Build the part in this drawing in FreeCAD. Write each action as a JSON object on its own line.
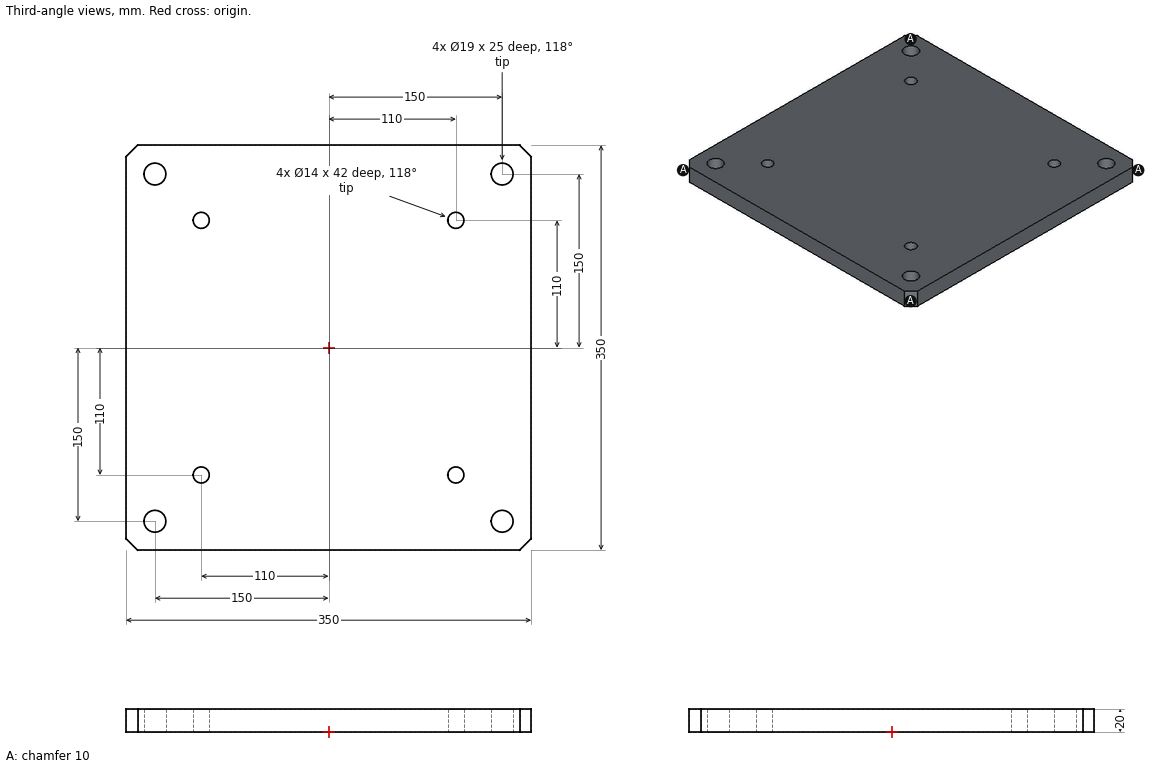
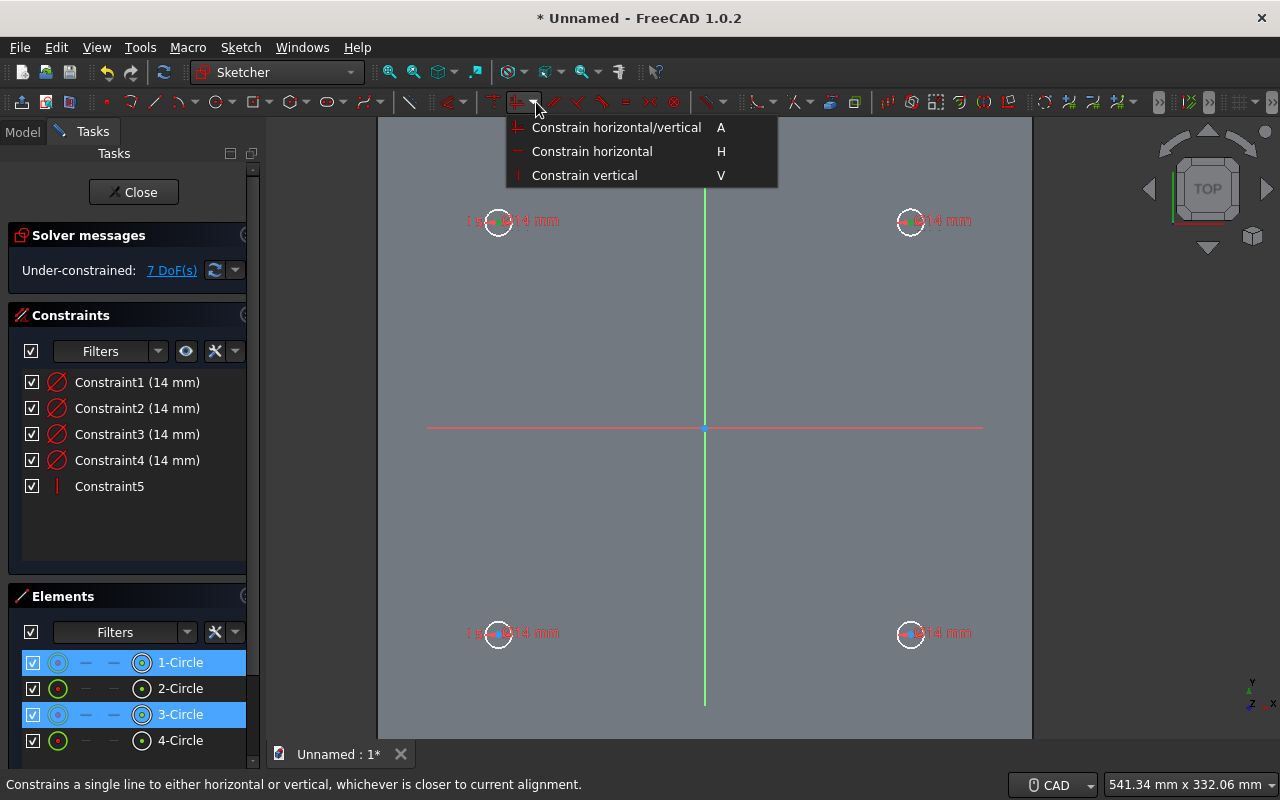
{"action": "left_click", "coordinate": [642, 151]}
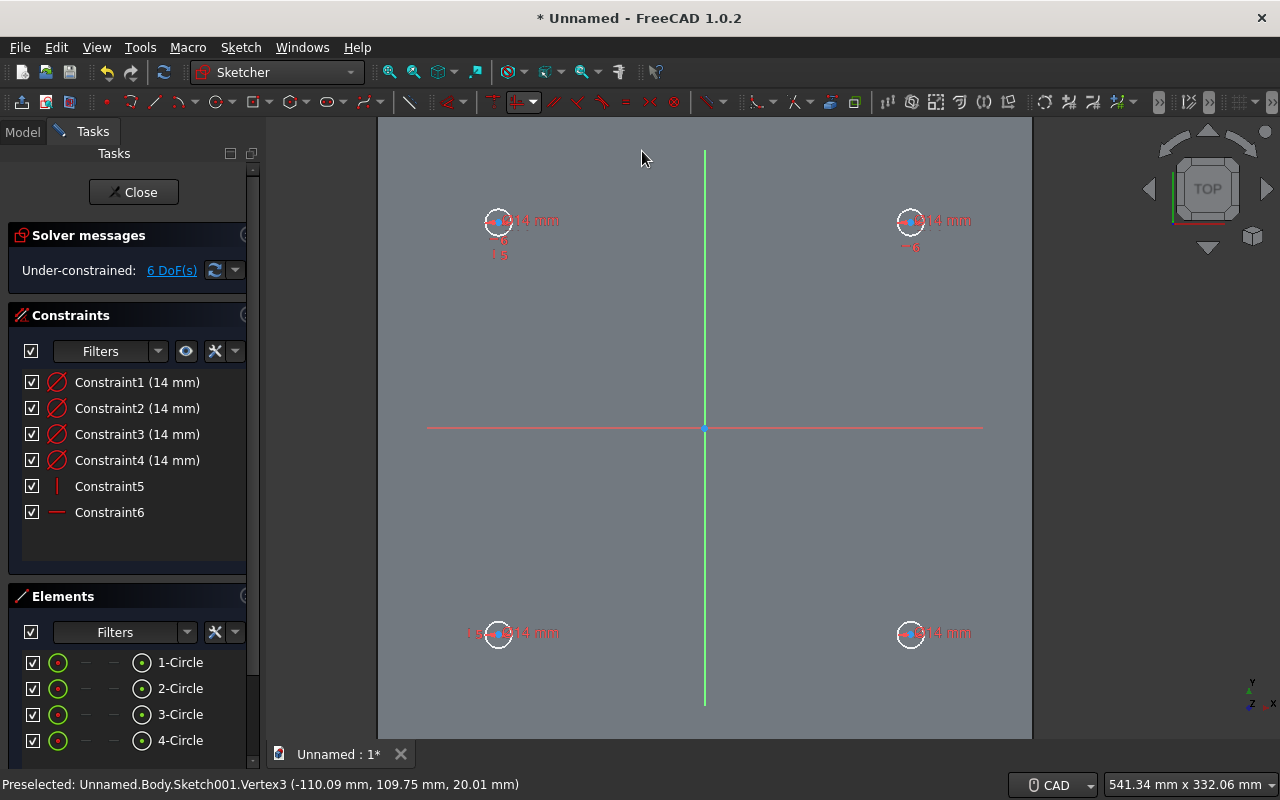
{"action": "left_click", "coordinate": [911, 223]}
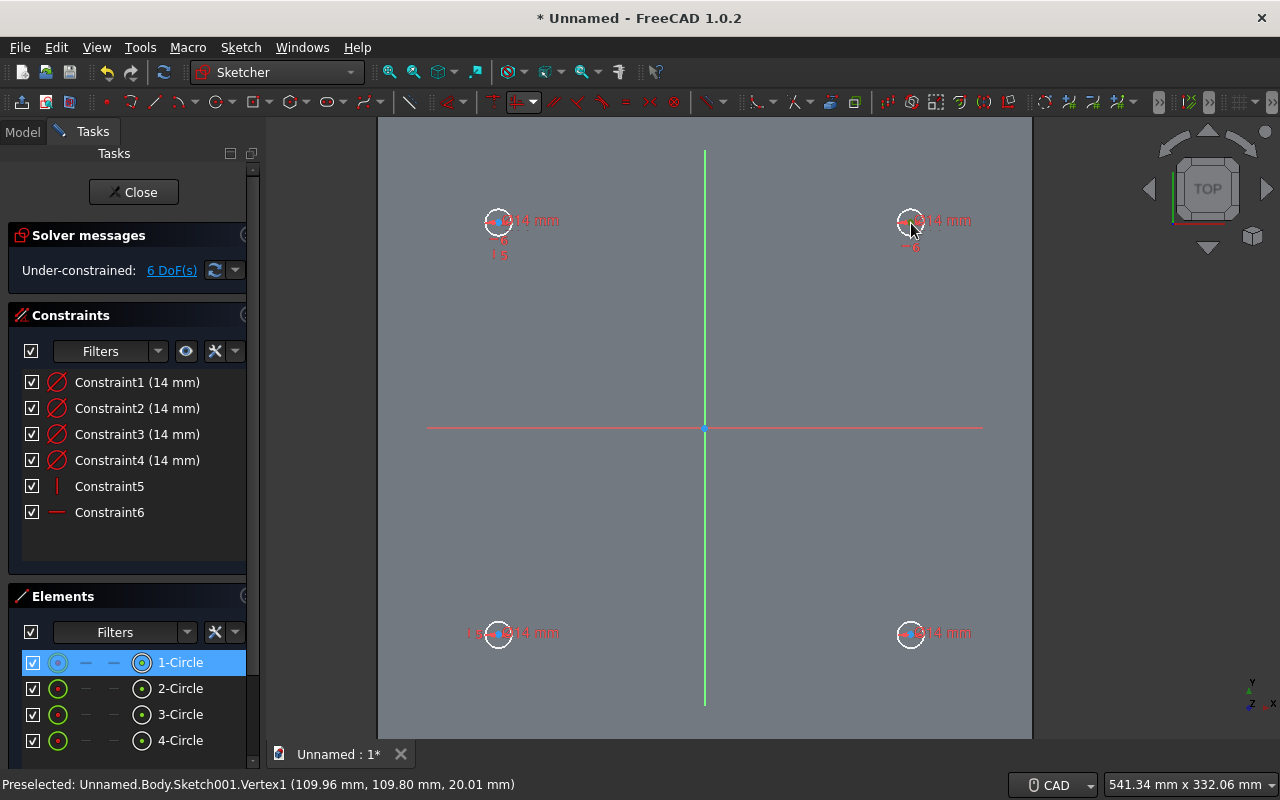
{"action": "left_click", "coordinate": [911, 635]}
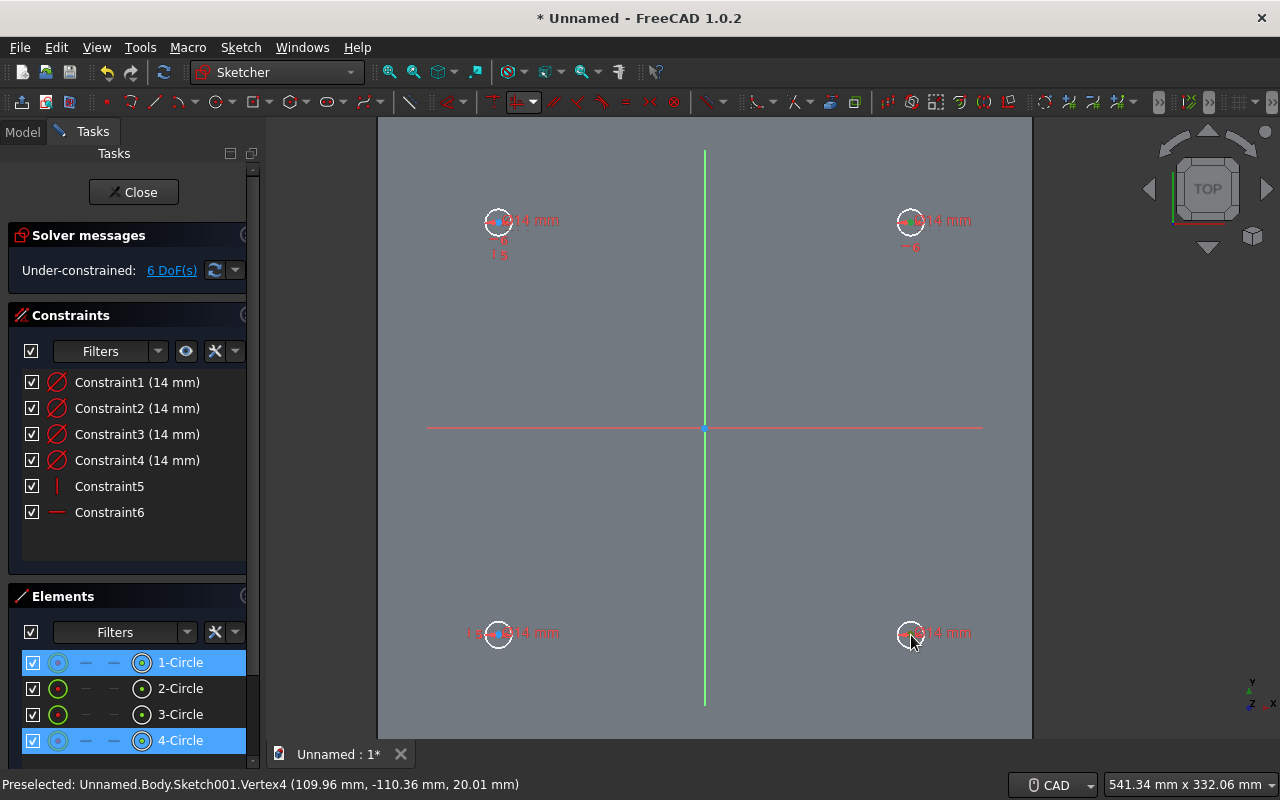
{"action": "key", "text": "v"}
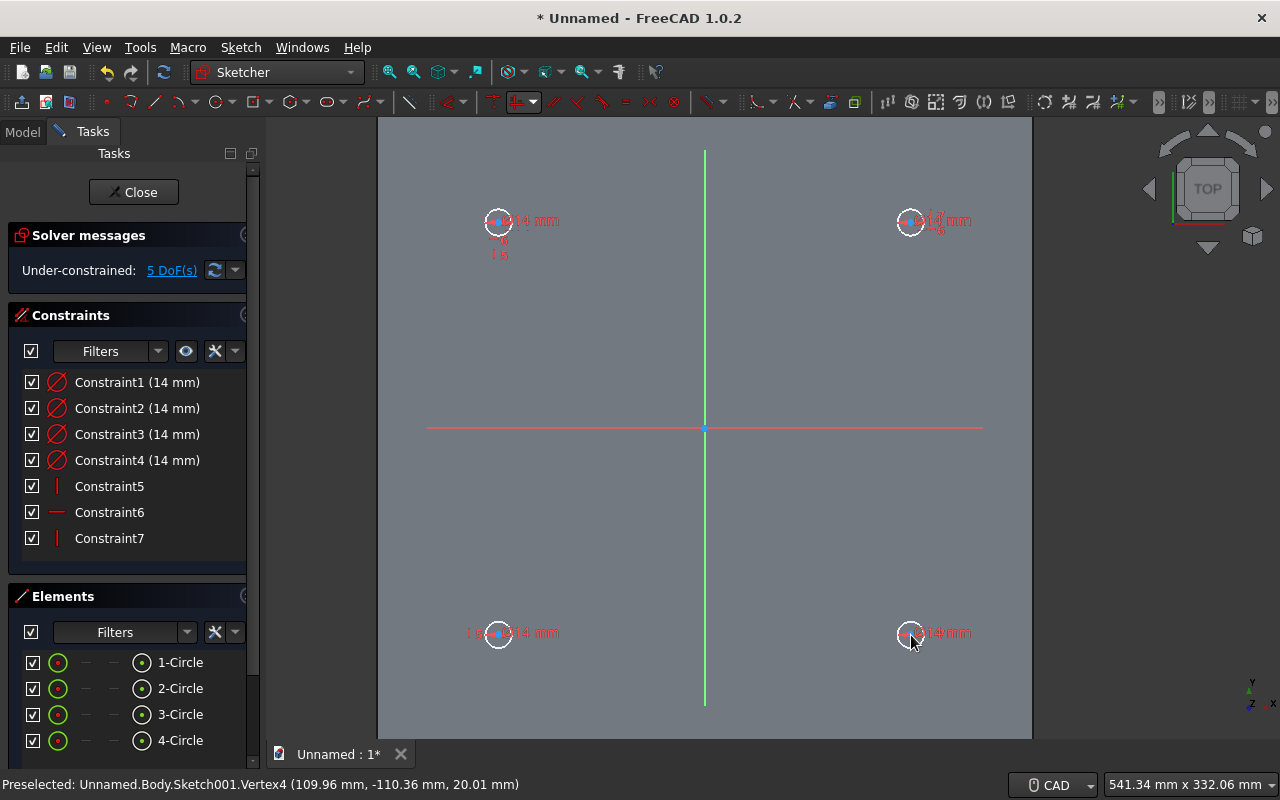
{"action": "left_click", "coordinate": [499, 635]}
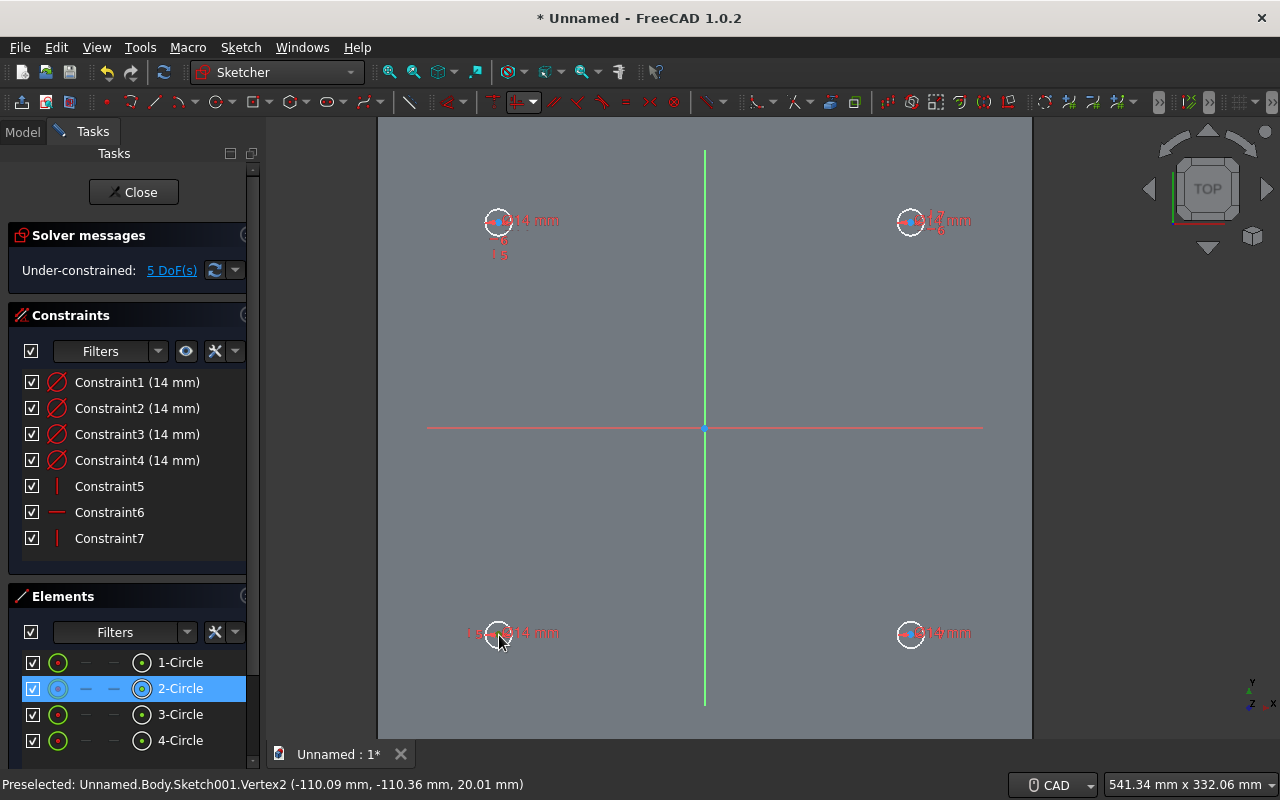
{"action": "left_click", "coordinate": [911, 635]}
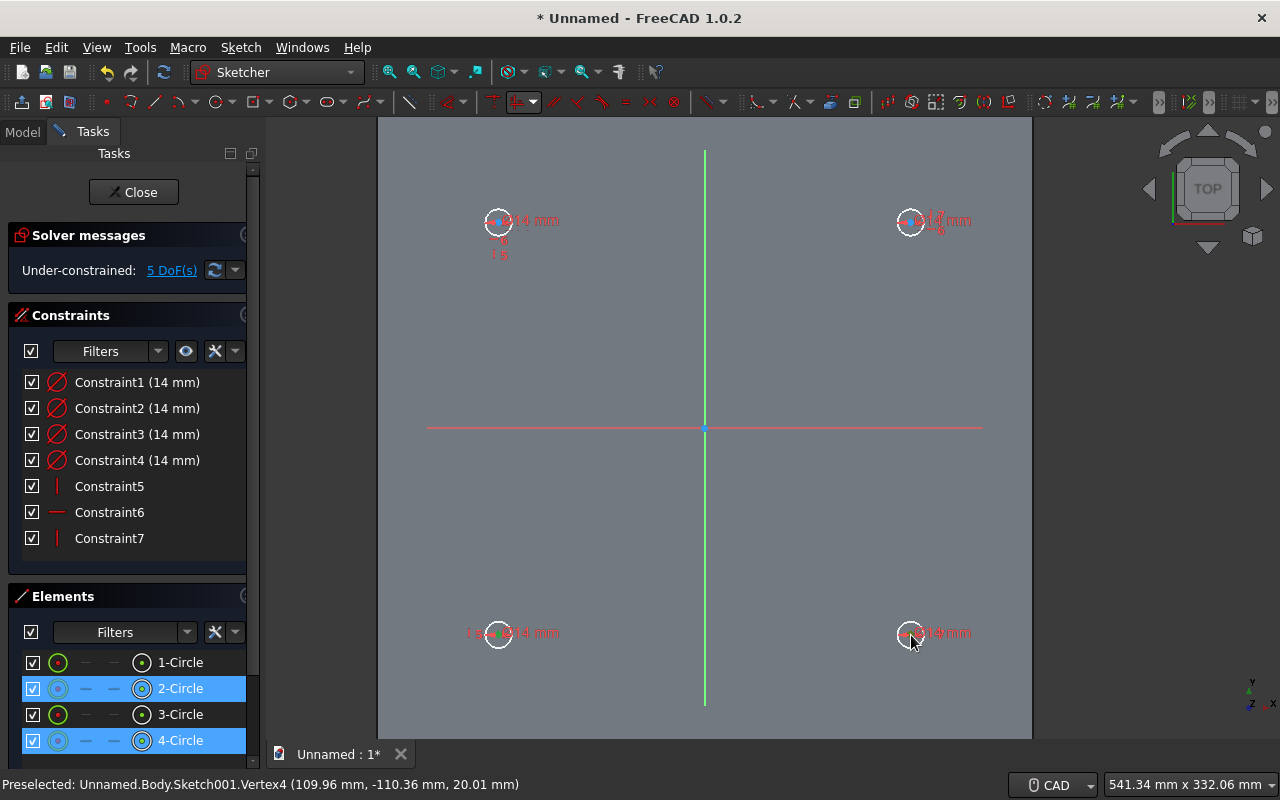
{"action": "key", "text": "h"}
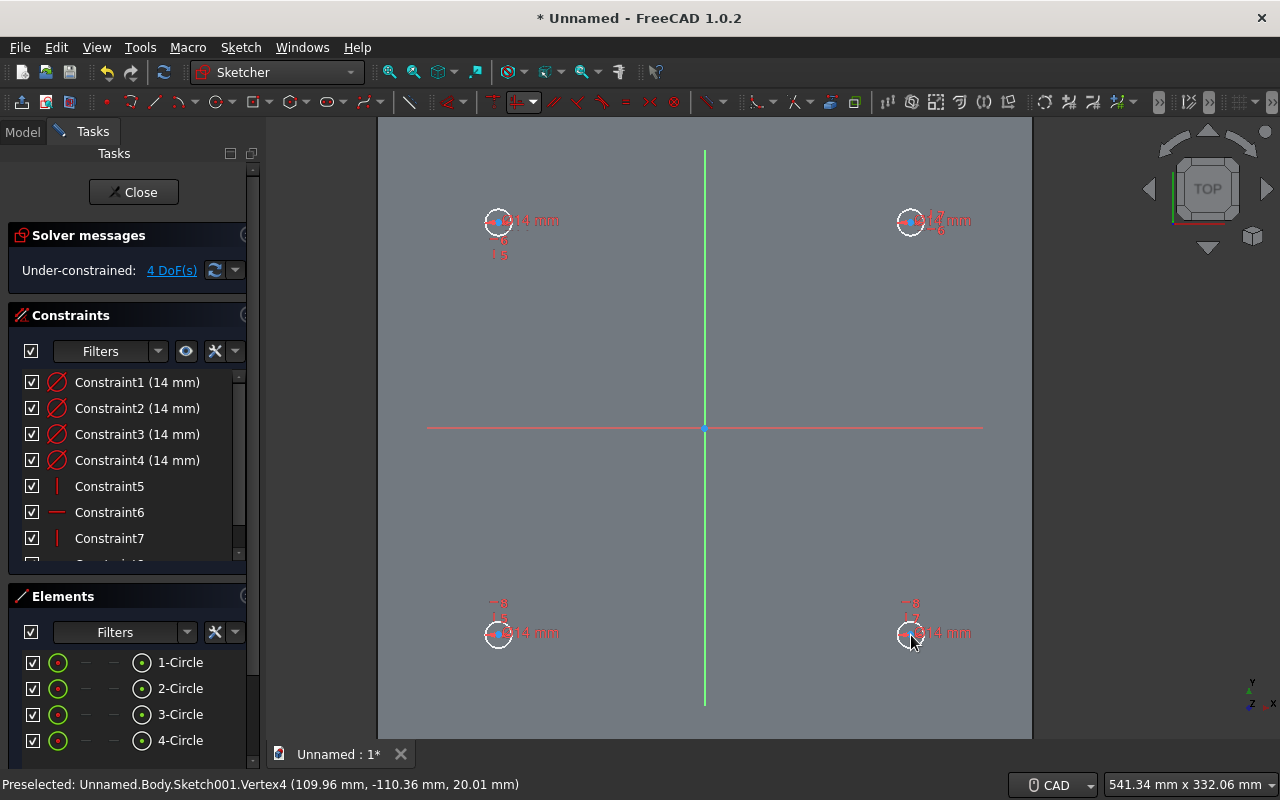
{"action": "left_click", "coordinate": [911, 223]}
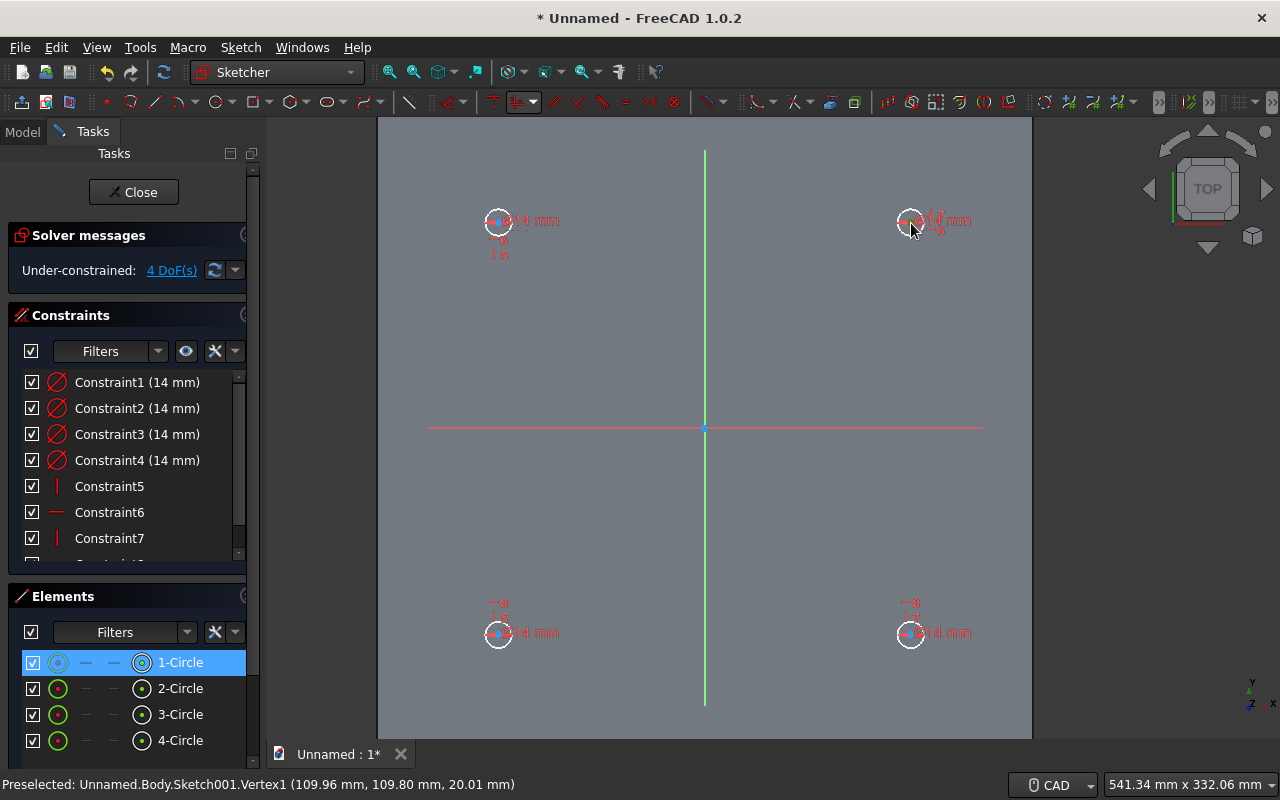
{"action": "left_click", "coordinate": [466, 102]}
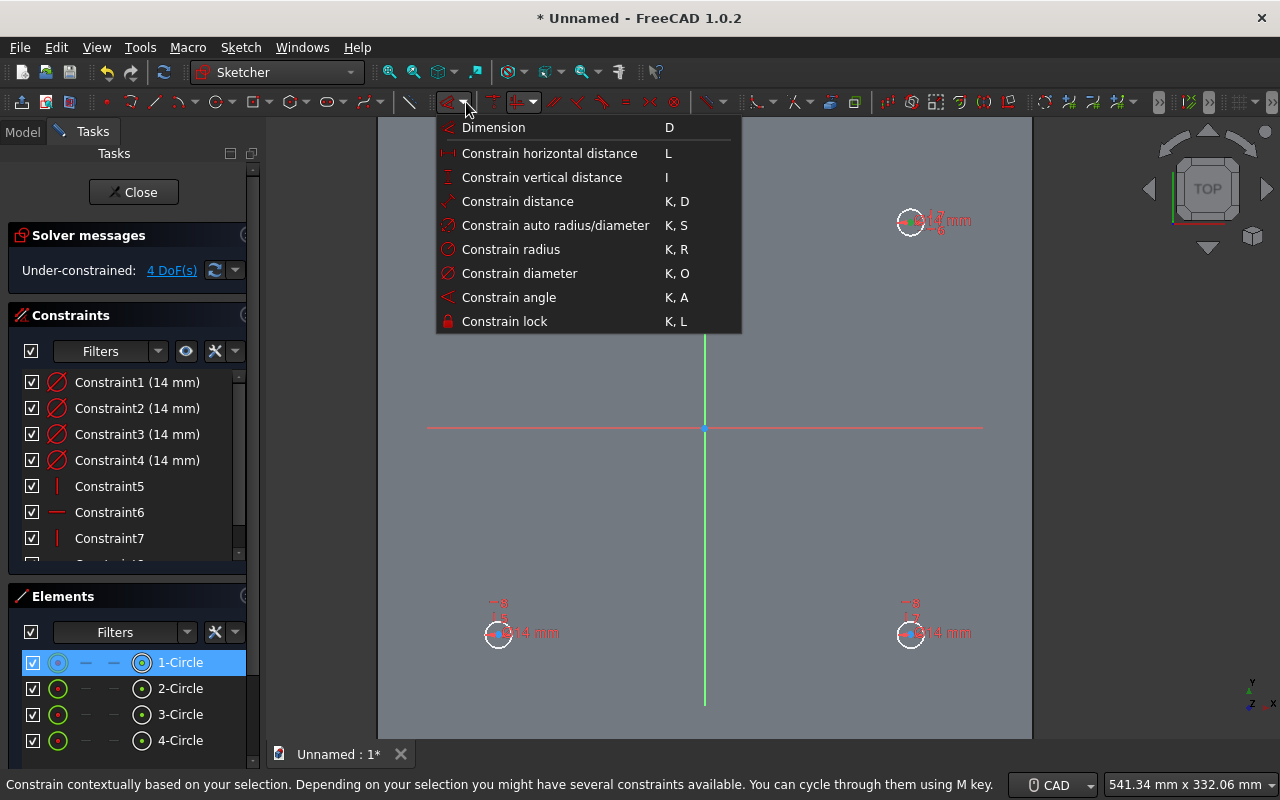
{"action": "left_click", "coordinate": [589, 153]}